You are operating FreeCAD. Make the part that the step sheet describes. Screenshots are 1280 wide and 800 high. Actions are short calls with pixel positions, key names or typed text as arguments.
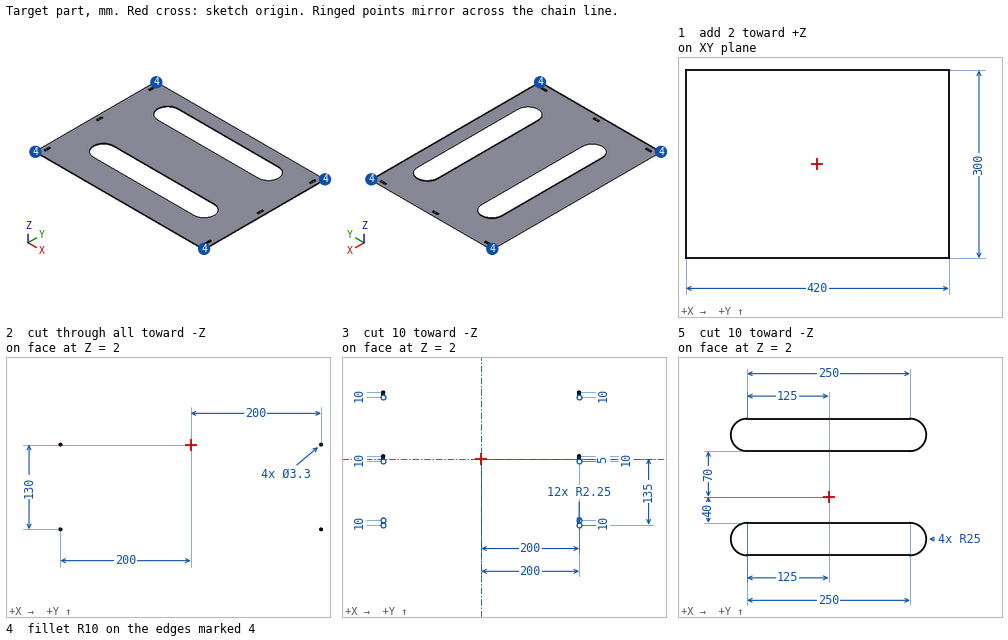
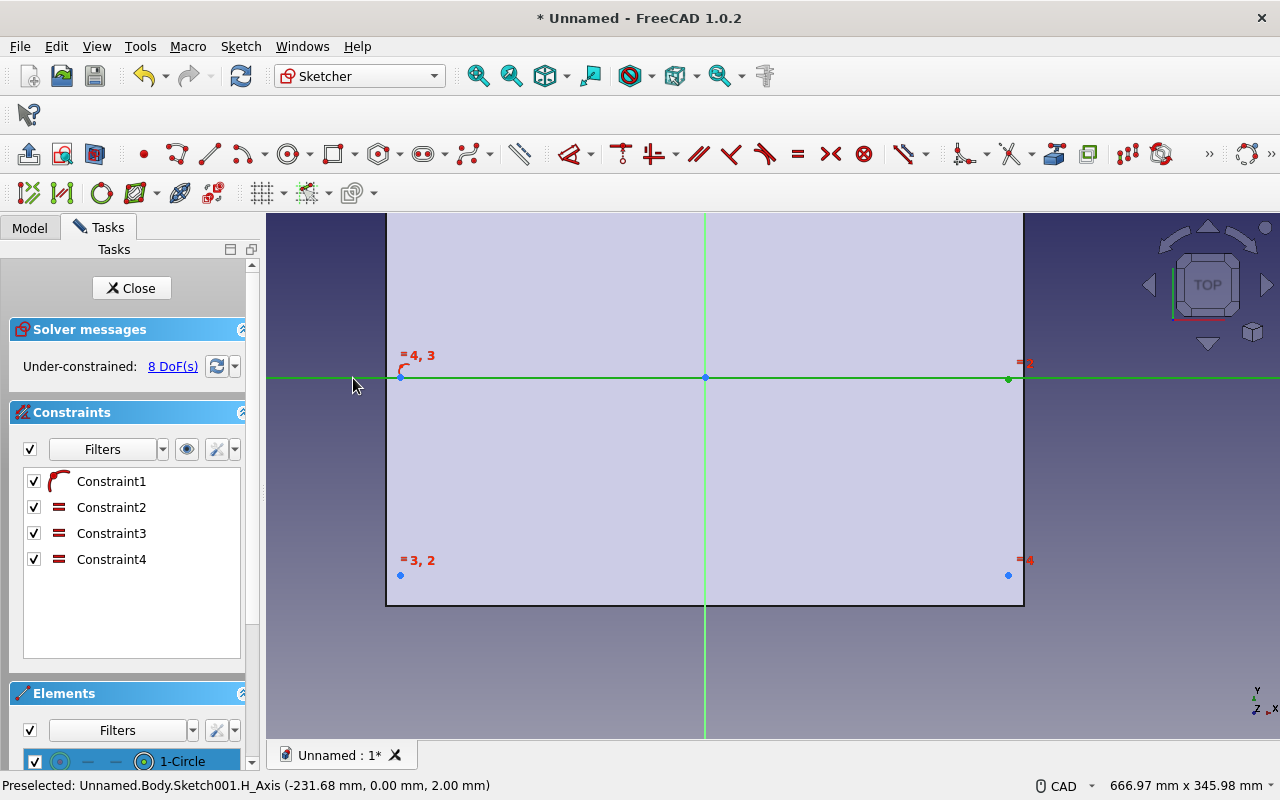
click(621, 154)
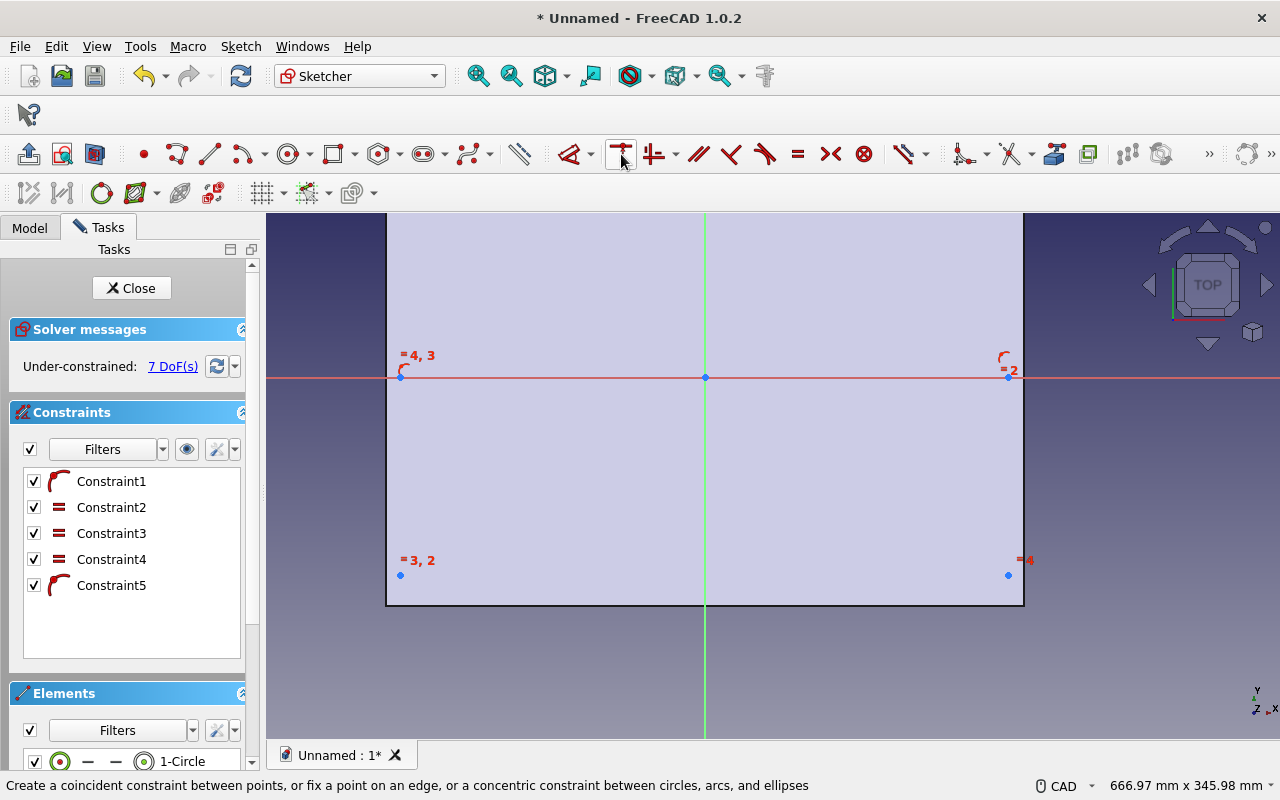
click(401, 576)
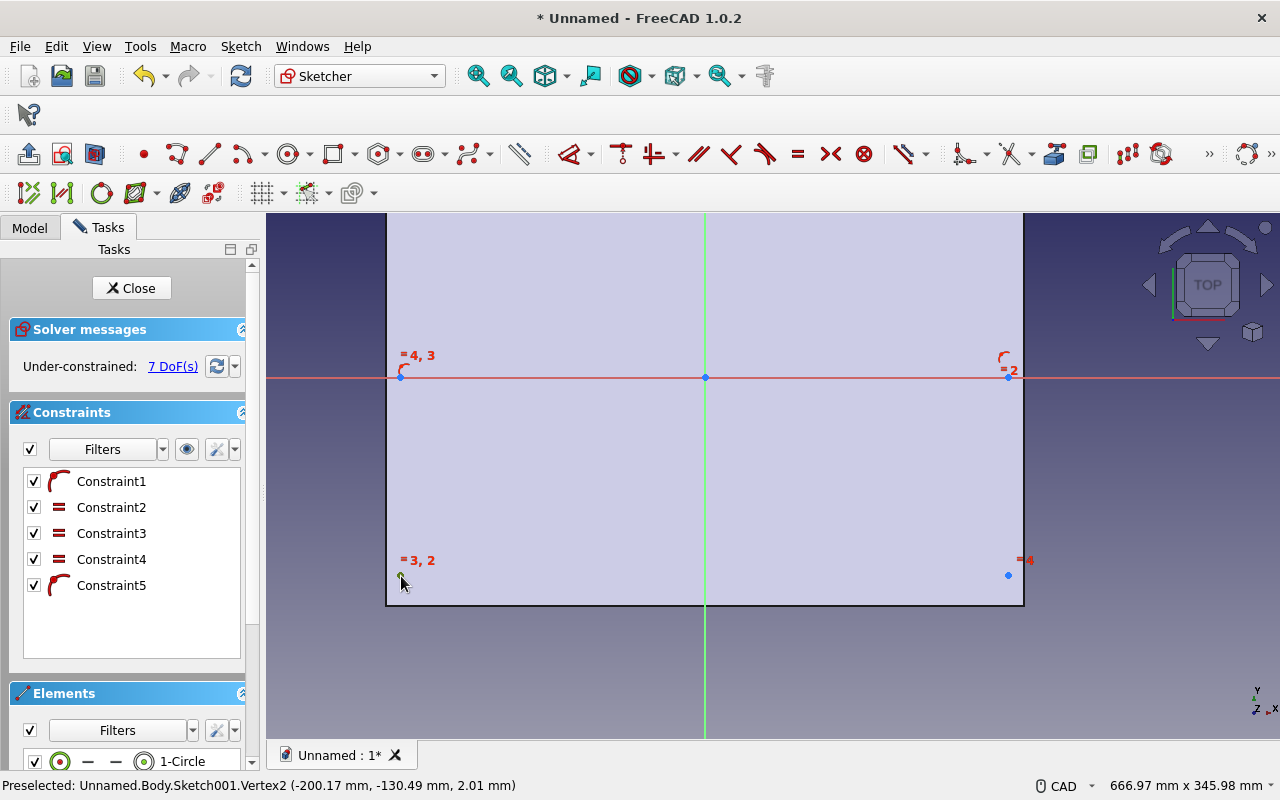
click(401, 378)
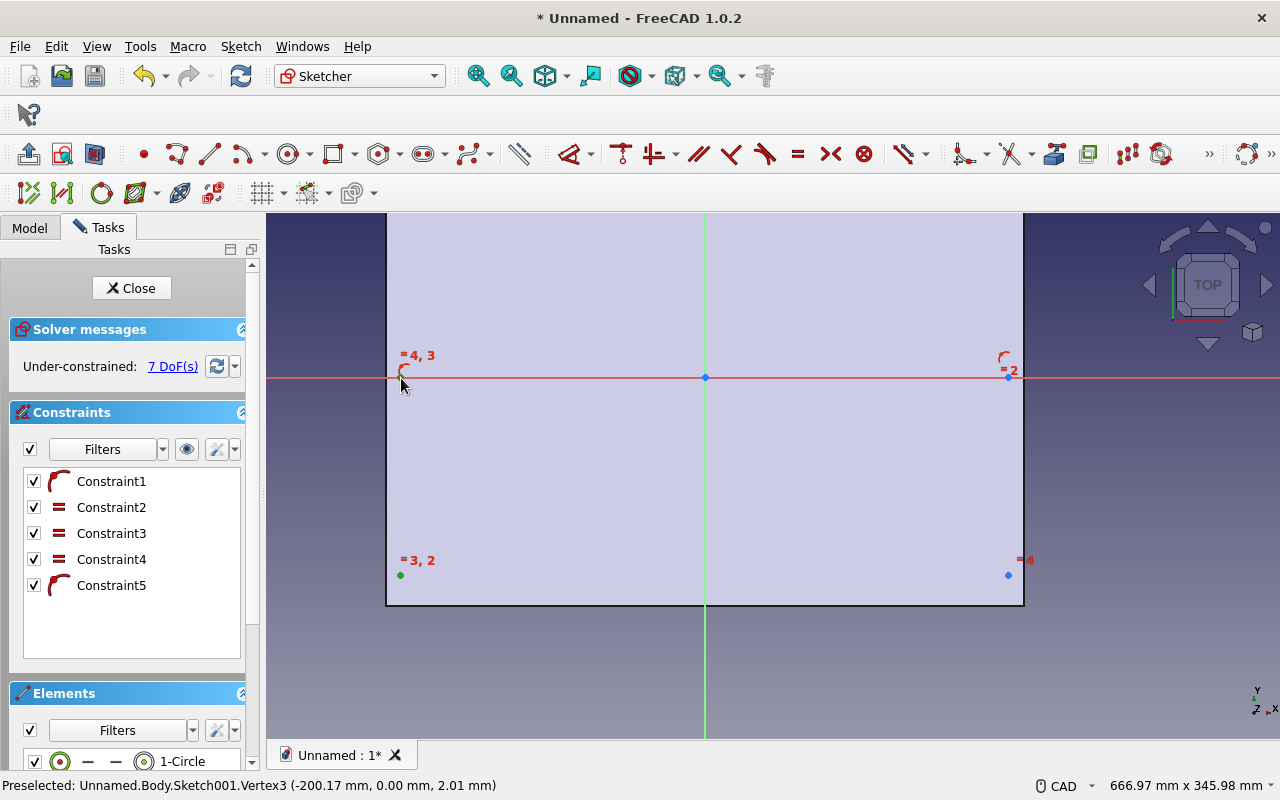
key(v)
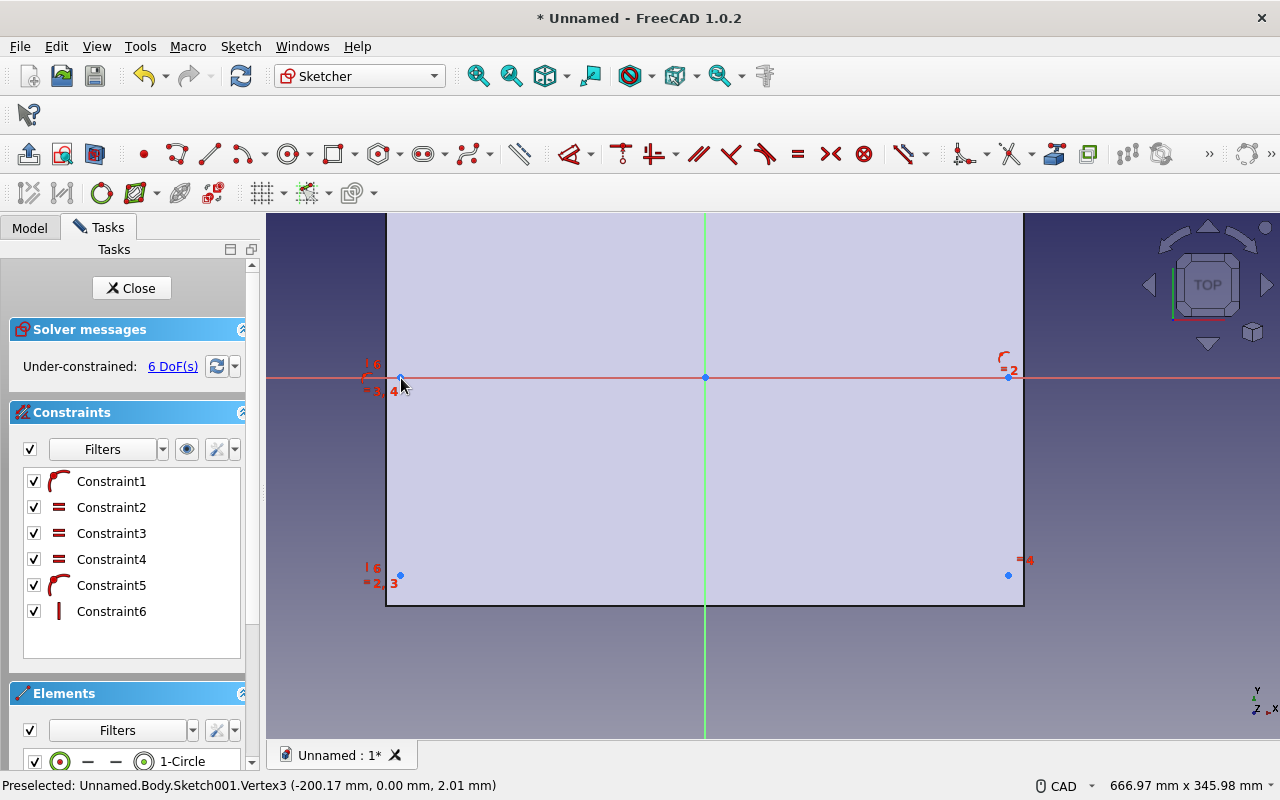
click(1009, 378)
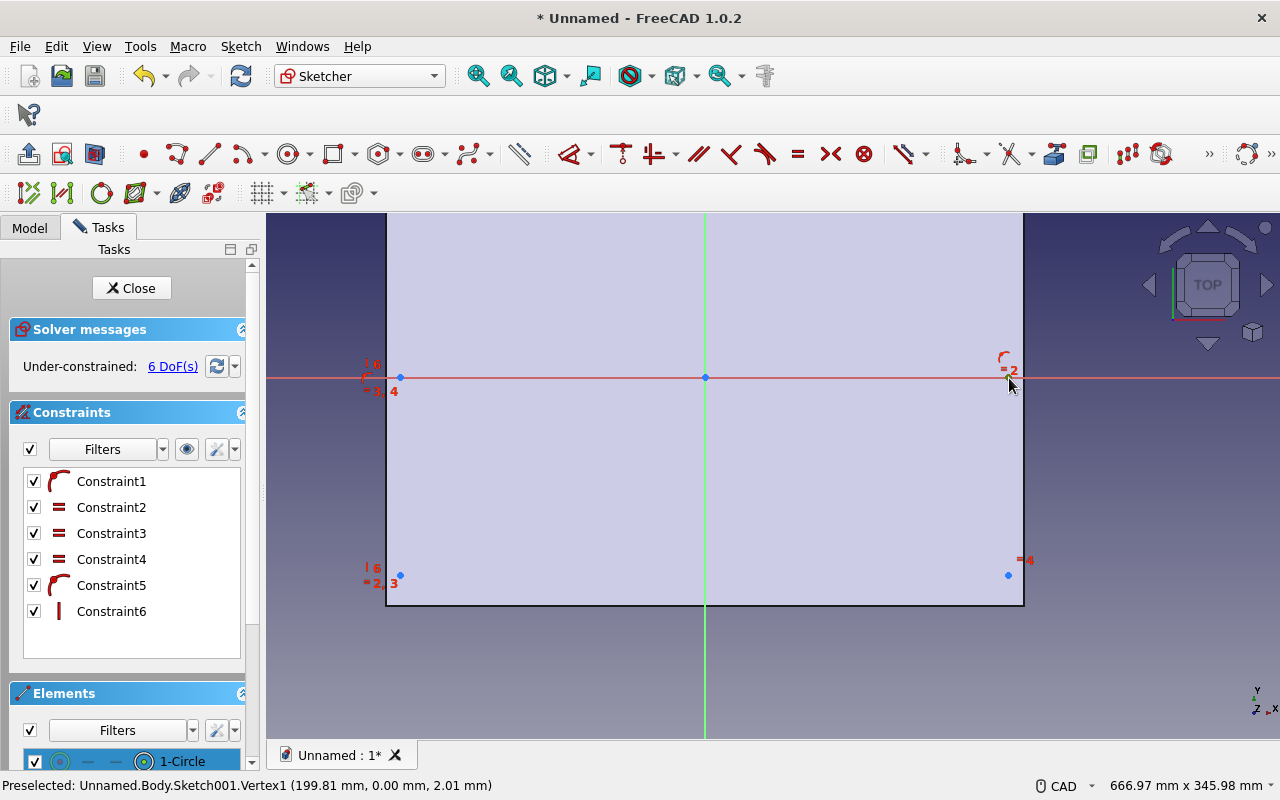
click(1009, 576)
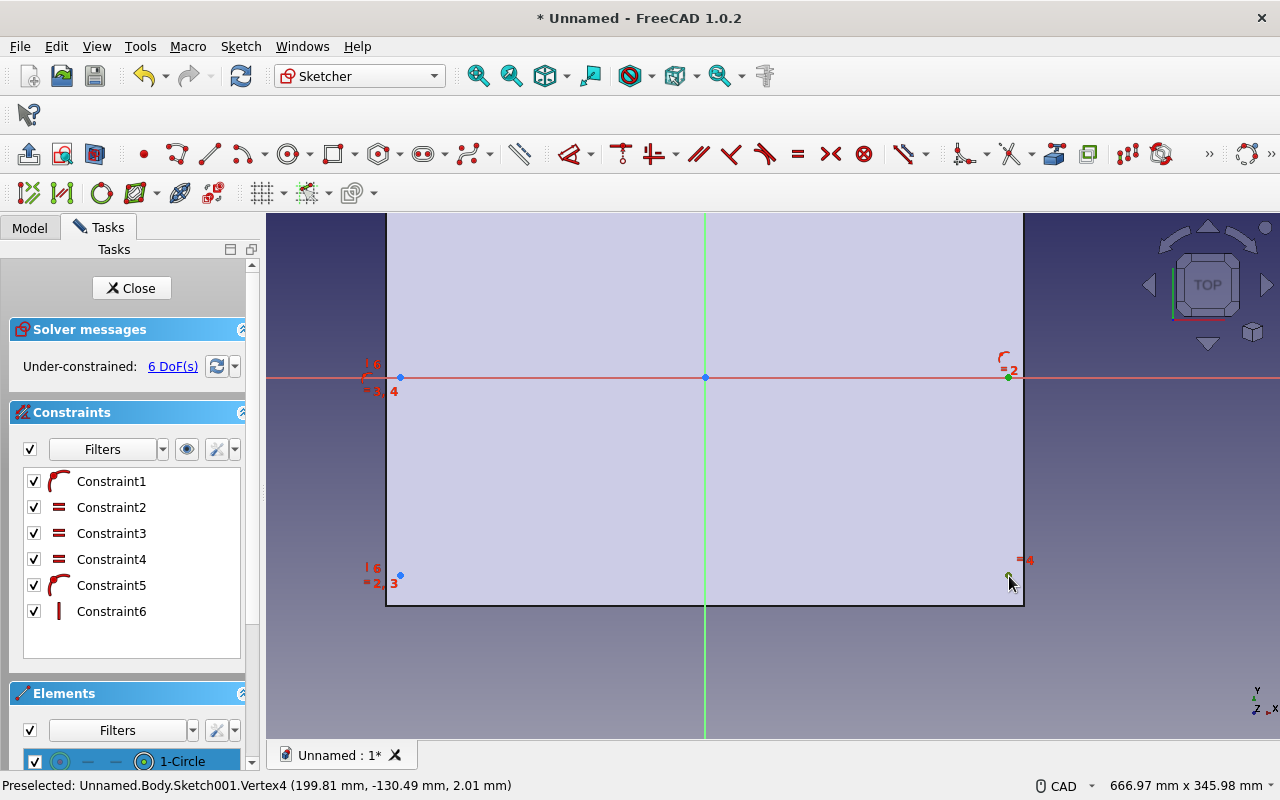
key(v)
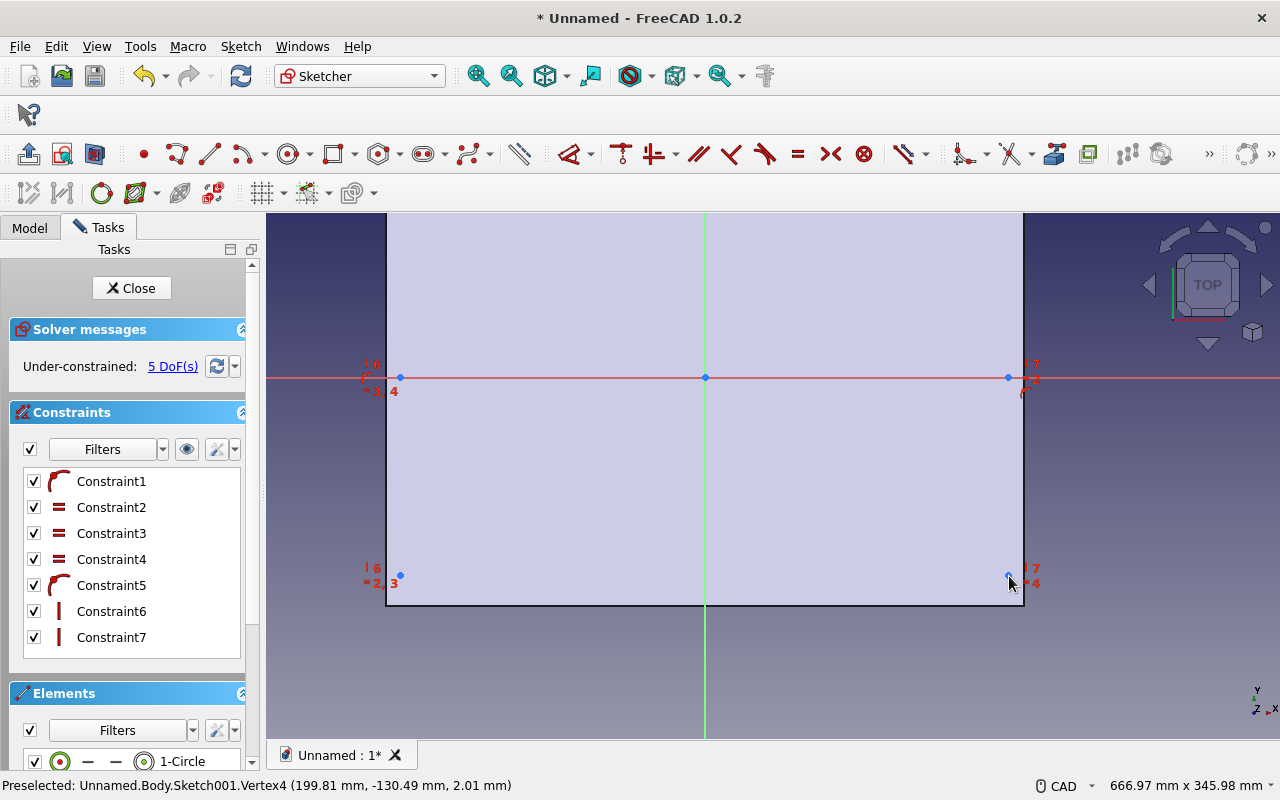
click(401, 576)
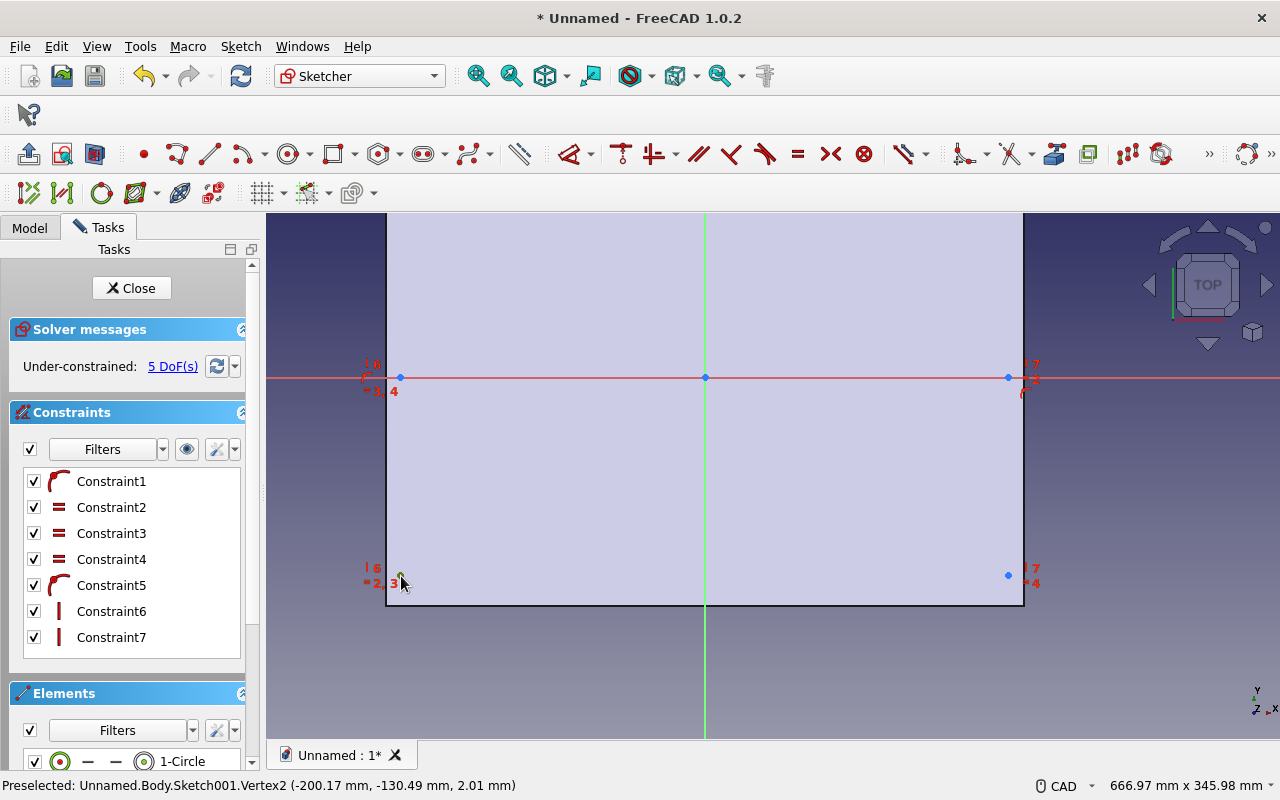
click(1009, 576)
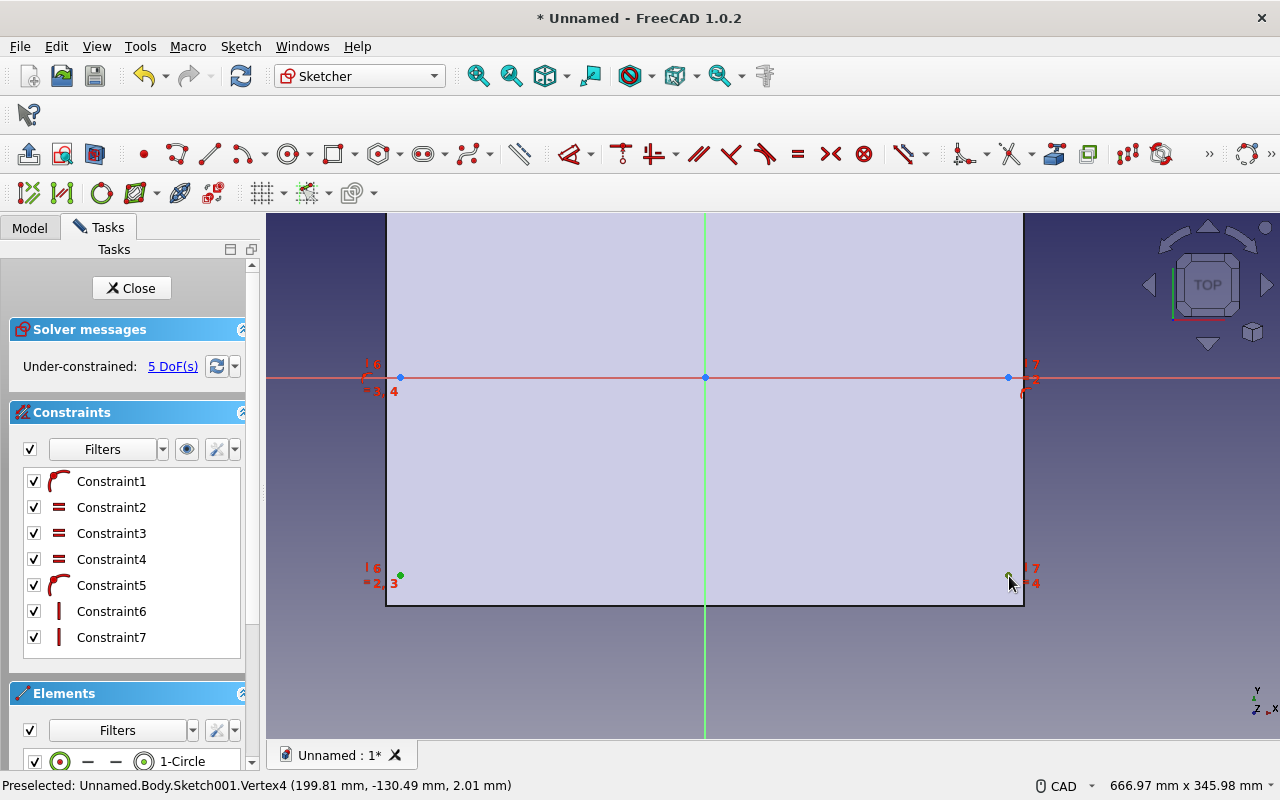
click(676, 154)